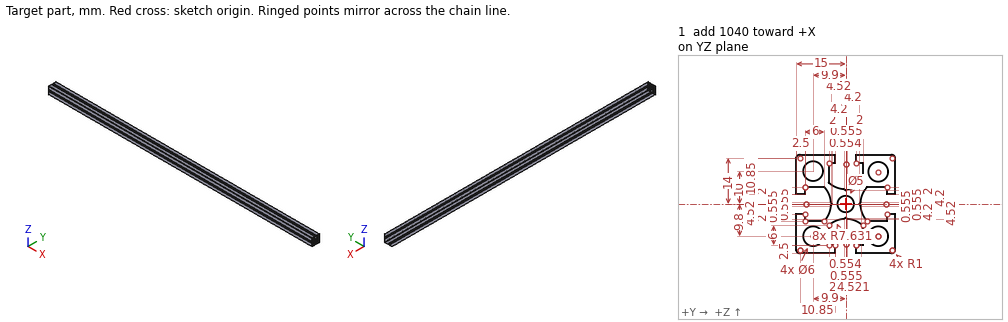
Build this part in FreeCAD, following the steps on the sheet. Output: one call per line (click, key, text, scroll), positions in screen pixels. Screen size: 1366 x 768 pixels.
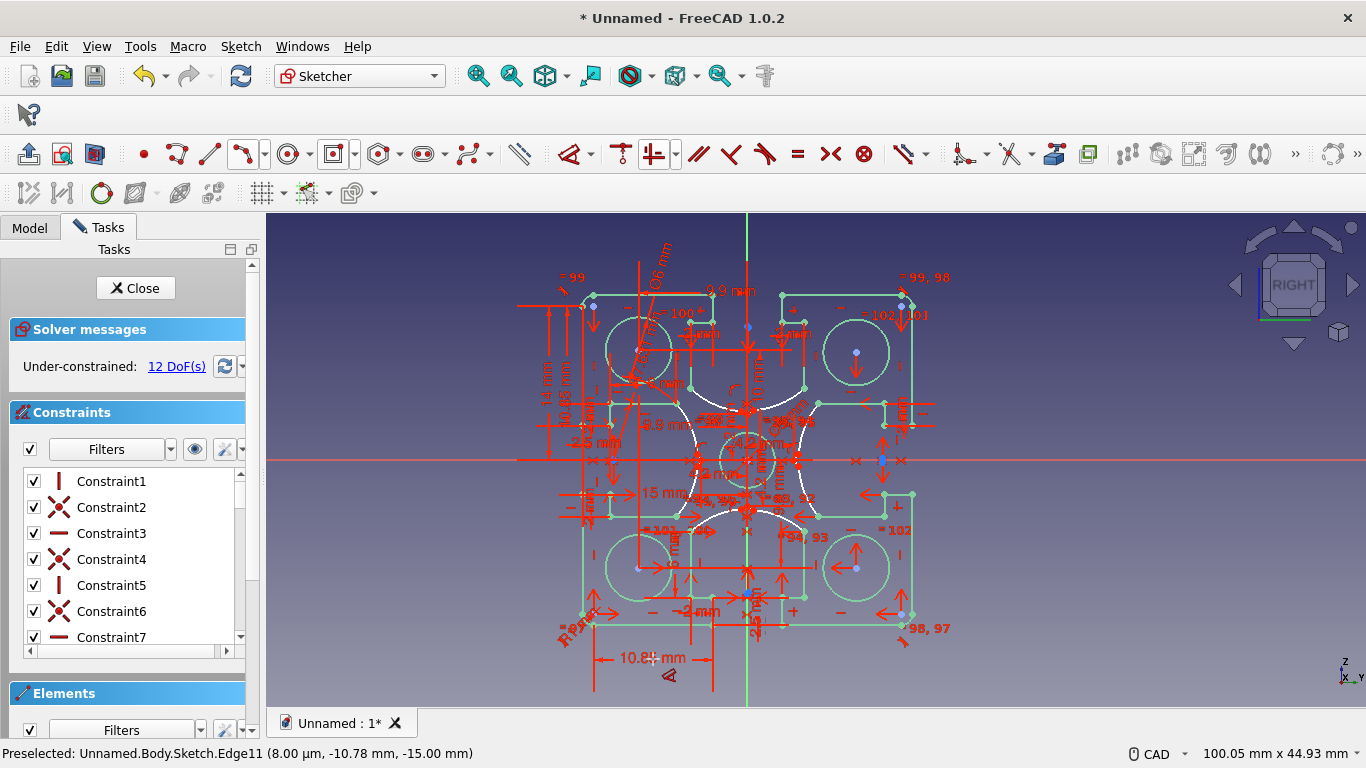
scroll(697, 454, up, 3)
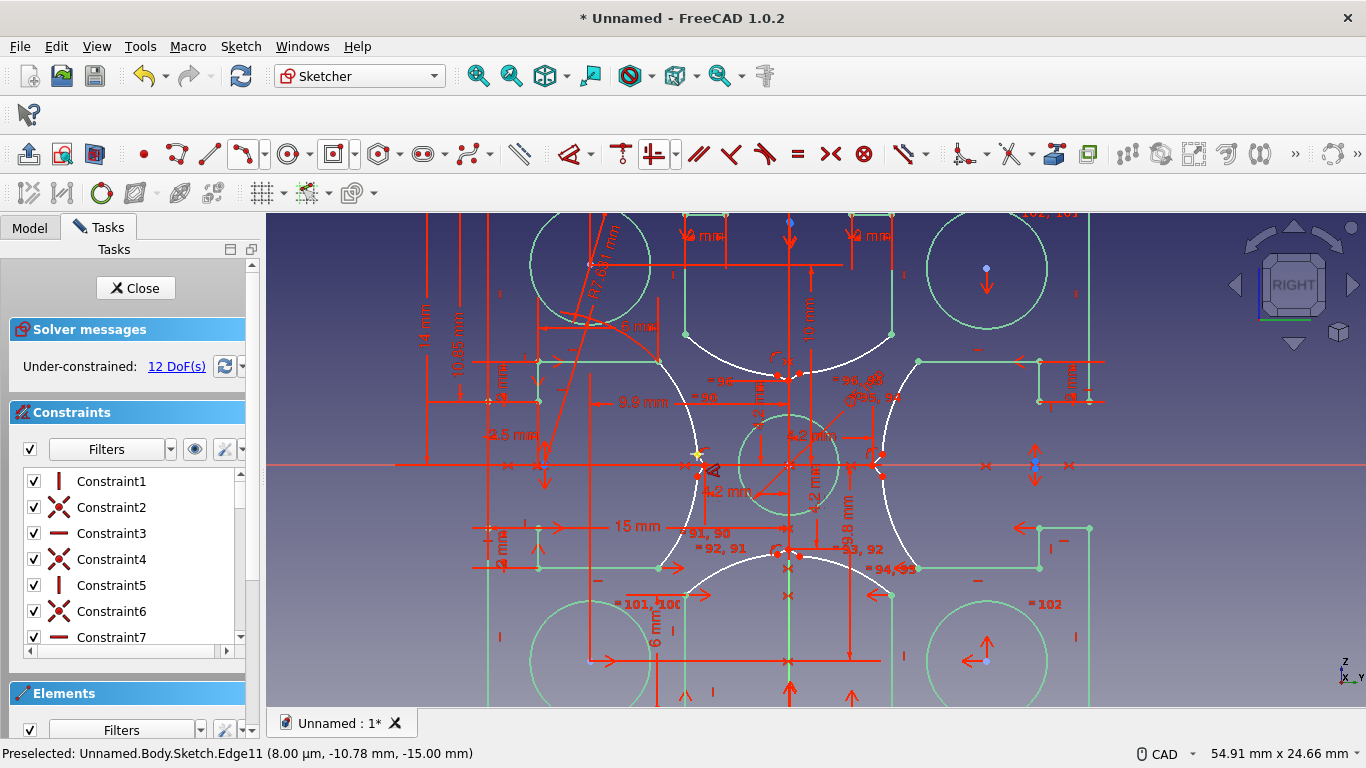
click(697, 454)
click(743, 523)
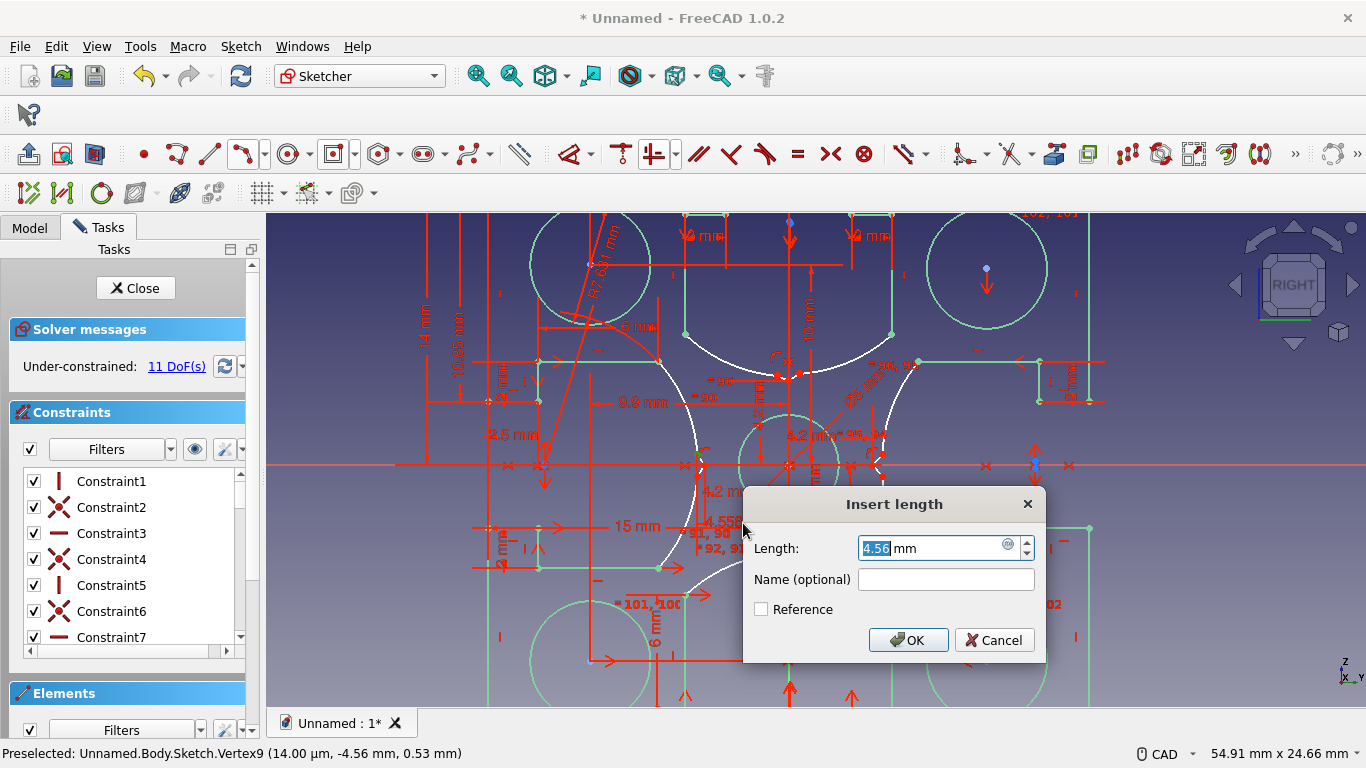
text(4.52)
key(Return)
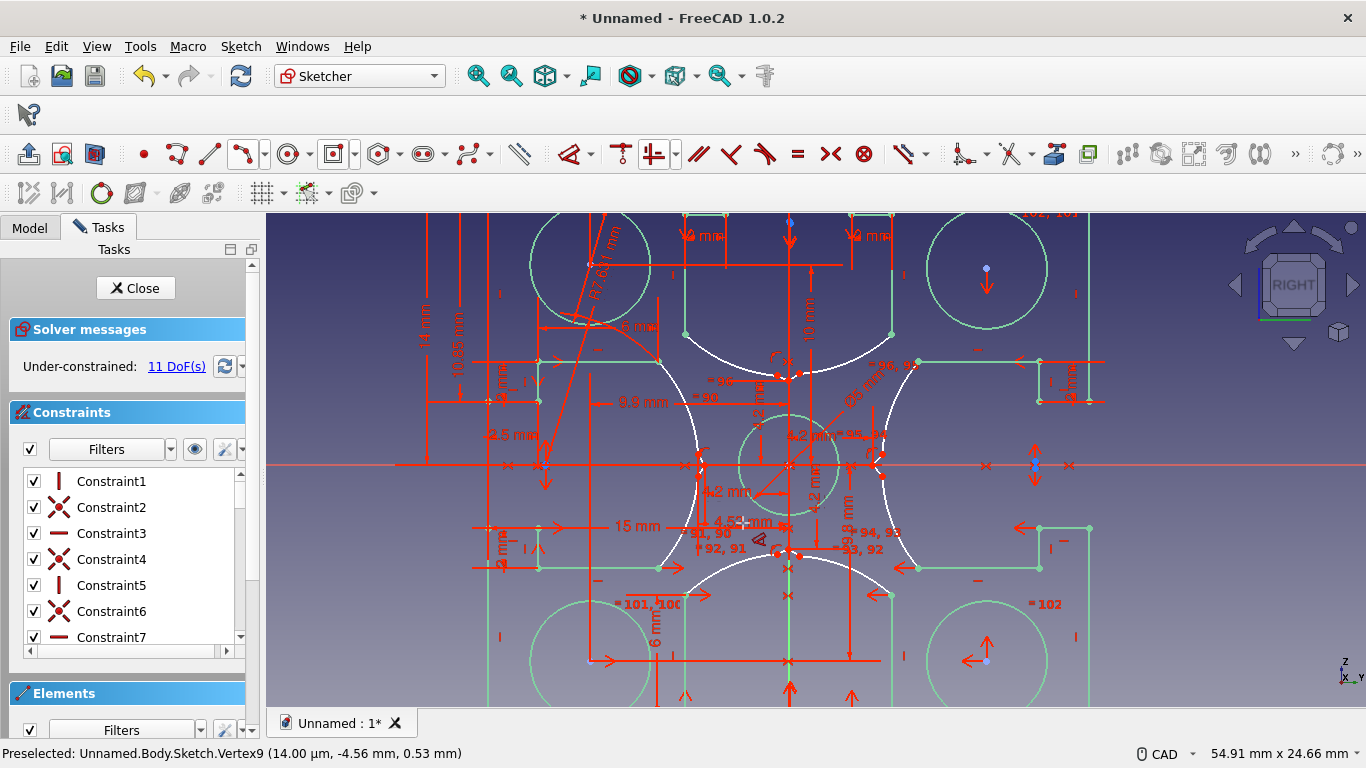
click(778, 554)
click(823, 541)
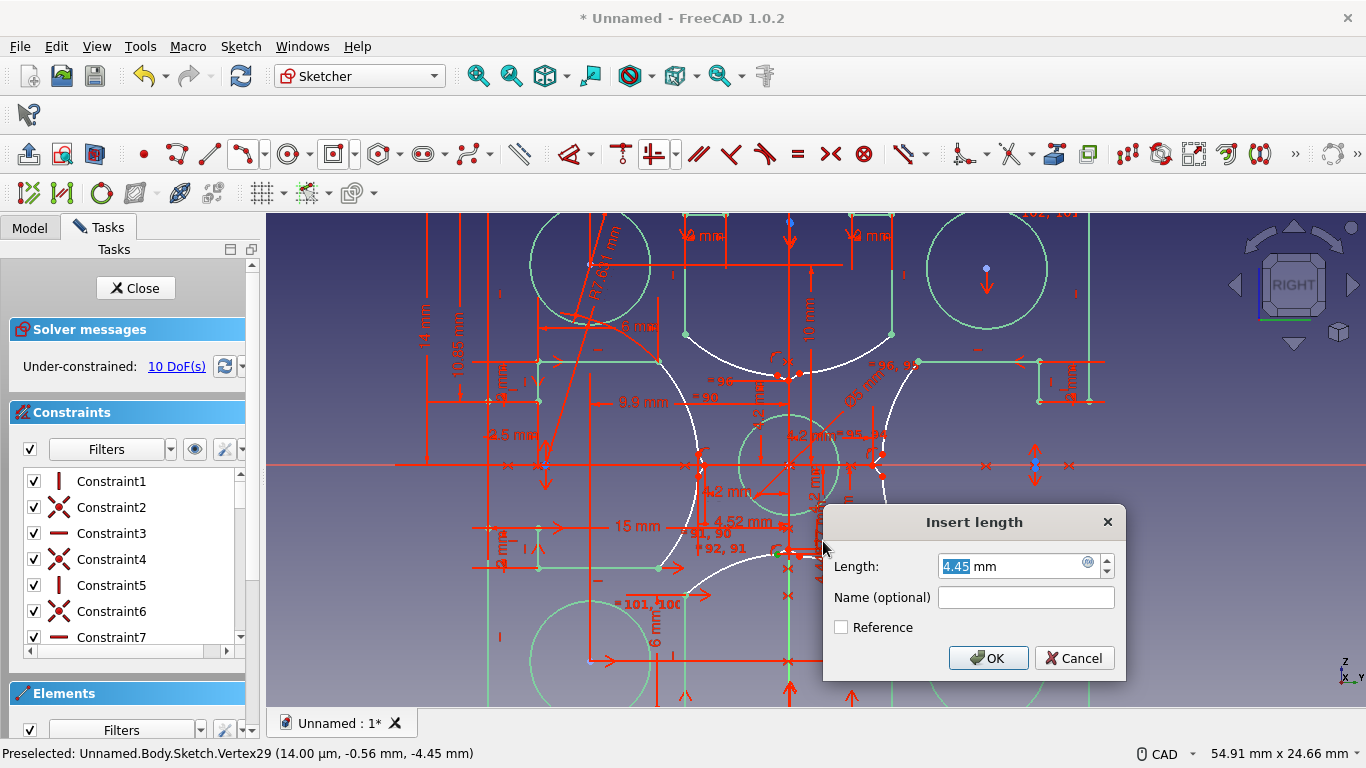
text(4.52)
key(Return)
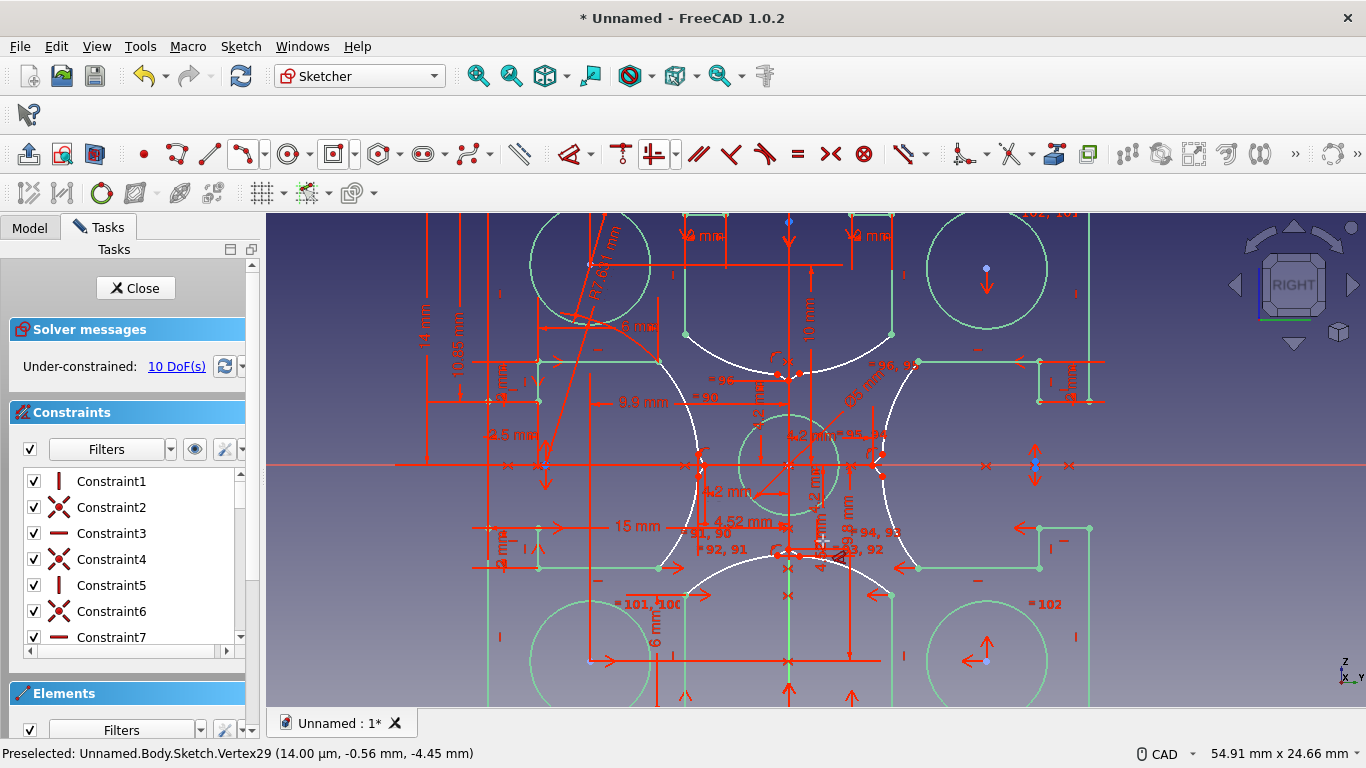
click(800, 556)
click(906, 490)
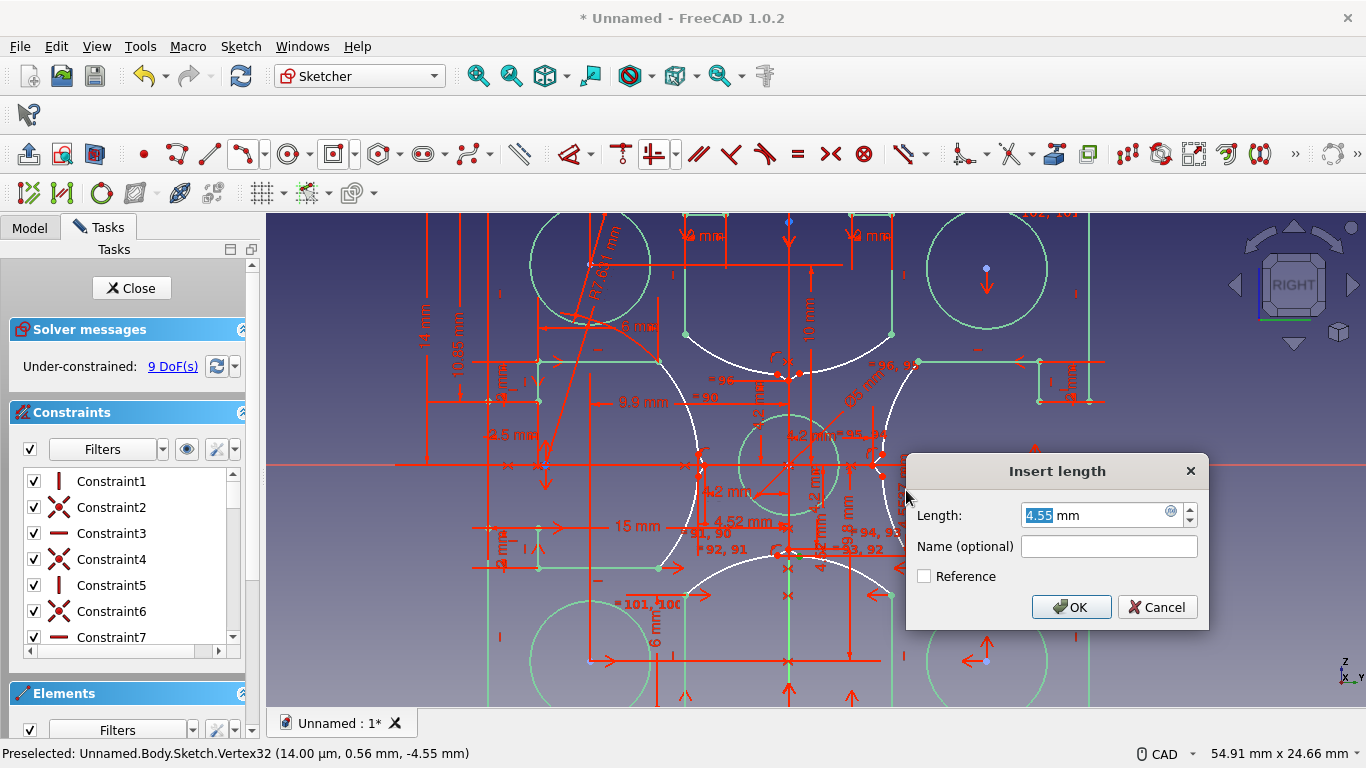
text(4.52)
key(Return)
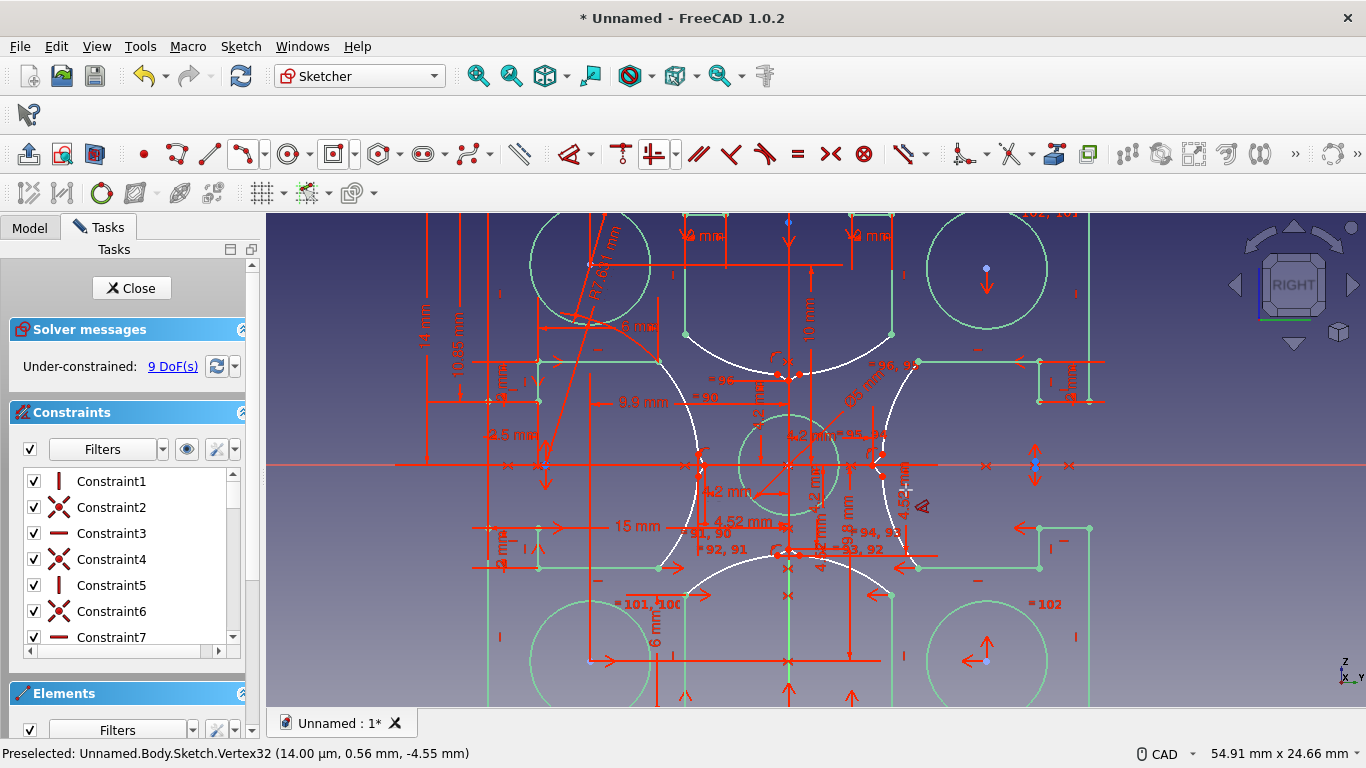
scroll(698, 454, up, 7)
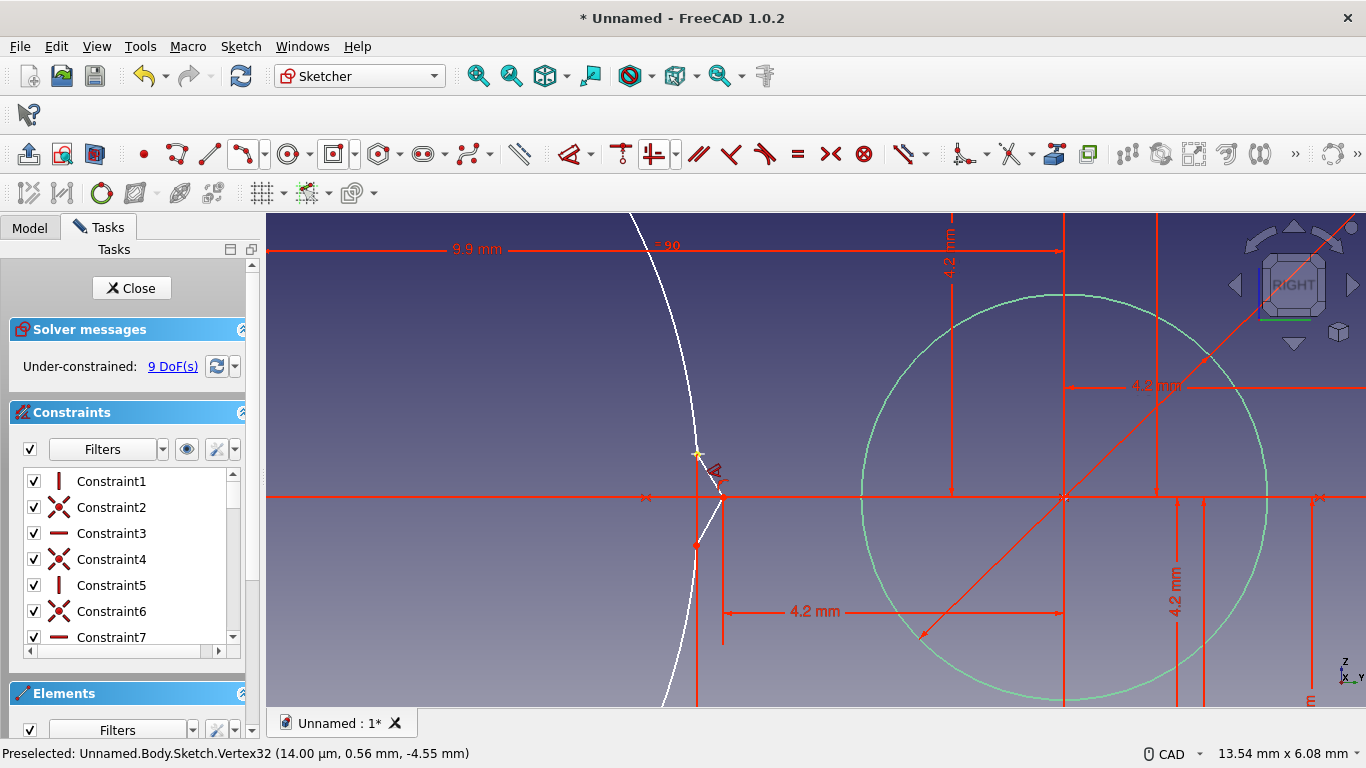
click(697, 454)
click(663, 476)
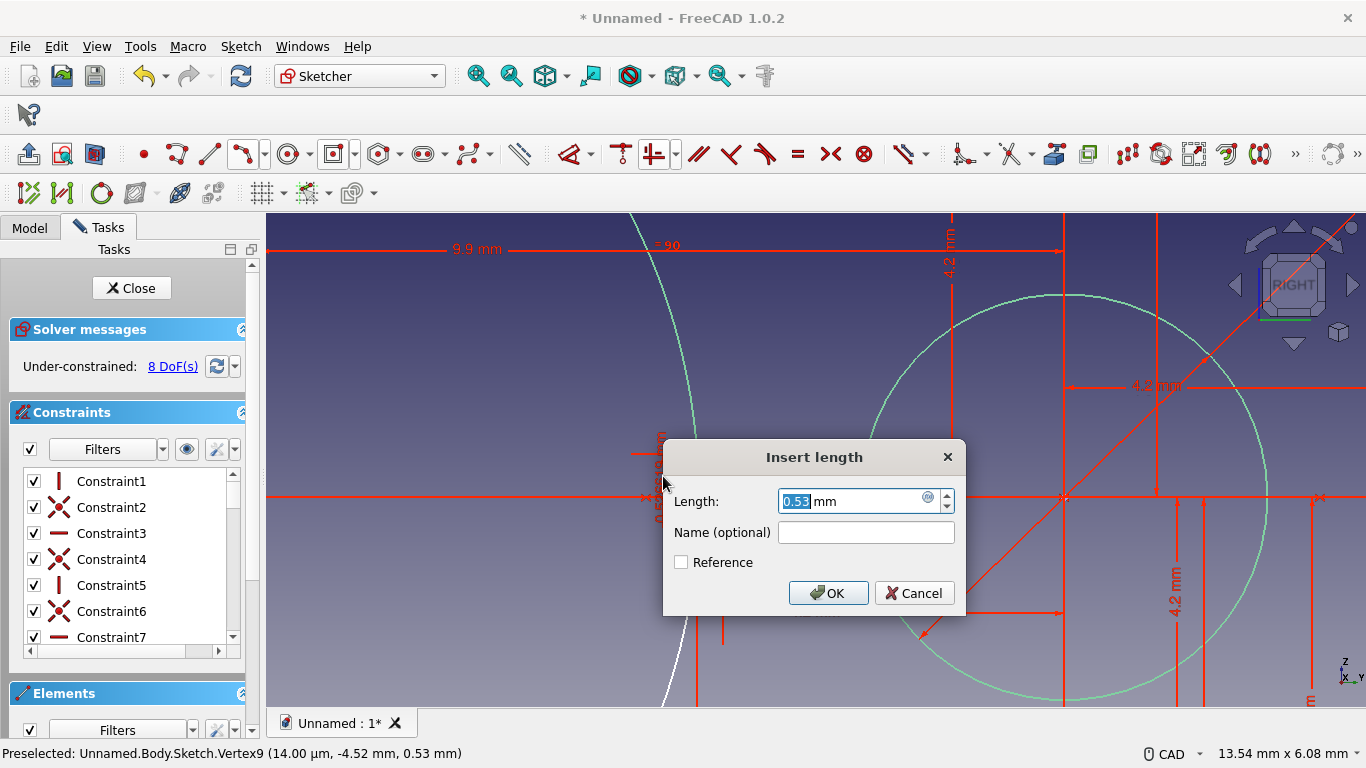
text(0.555)
key(Return)